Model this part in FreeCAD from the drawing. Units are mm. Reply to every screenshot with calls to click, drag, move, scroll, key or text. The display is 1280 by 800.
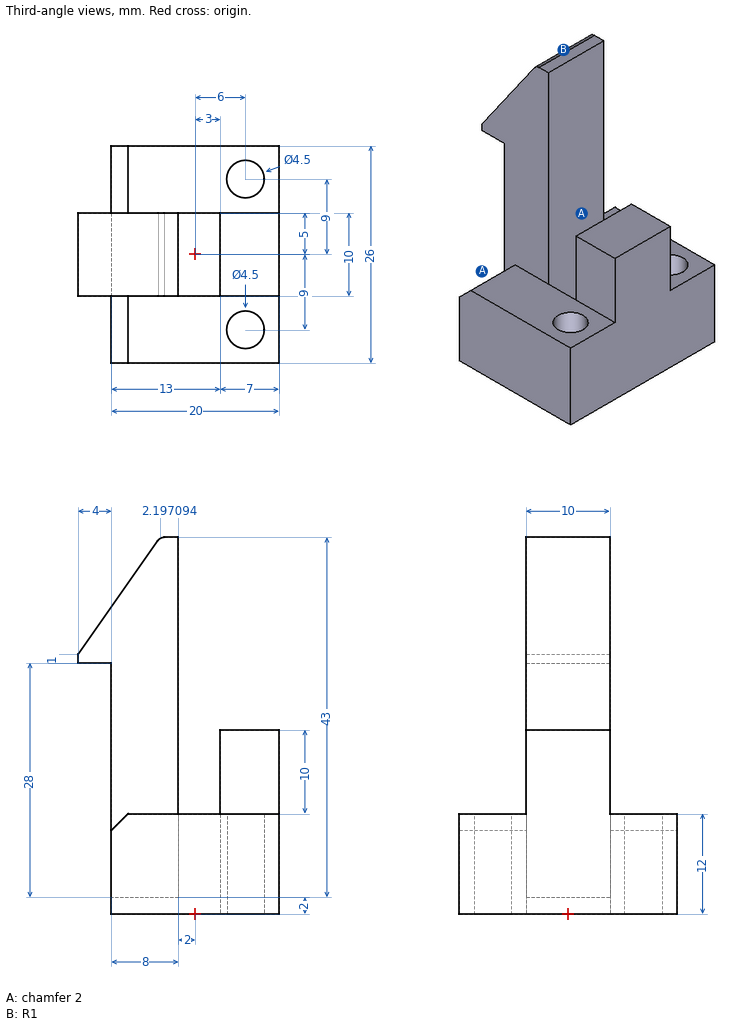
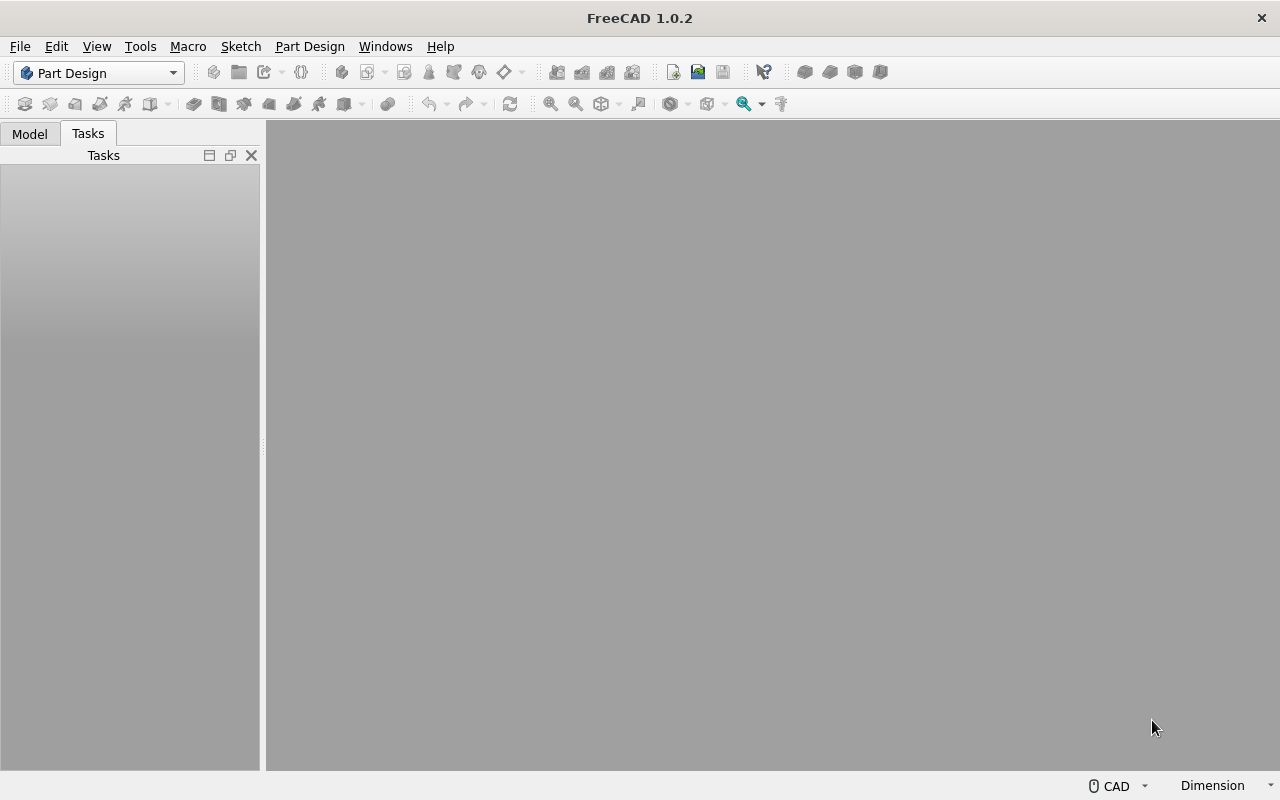
key(ctrl+n)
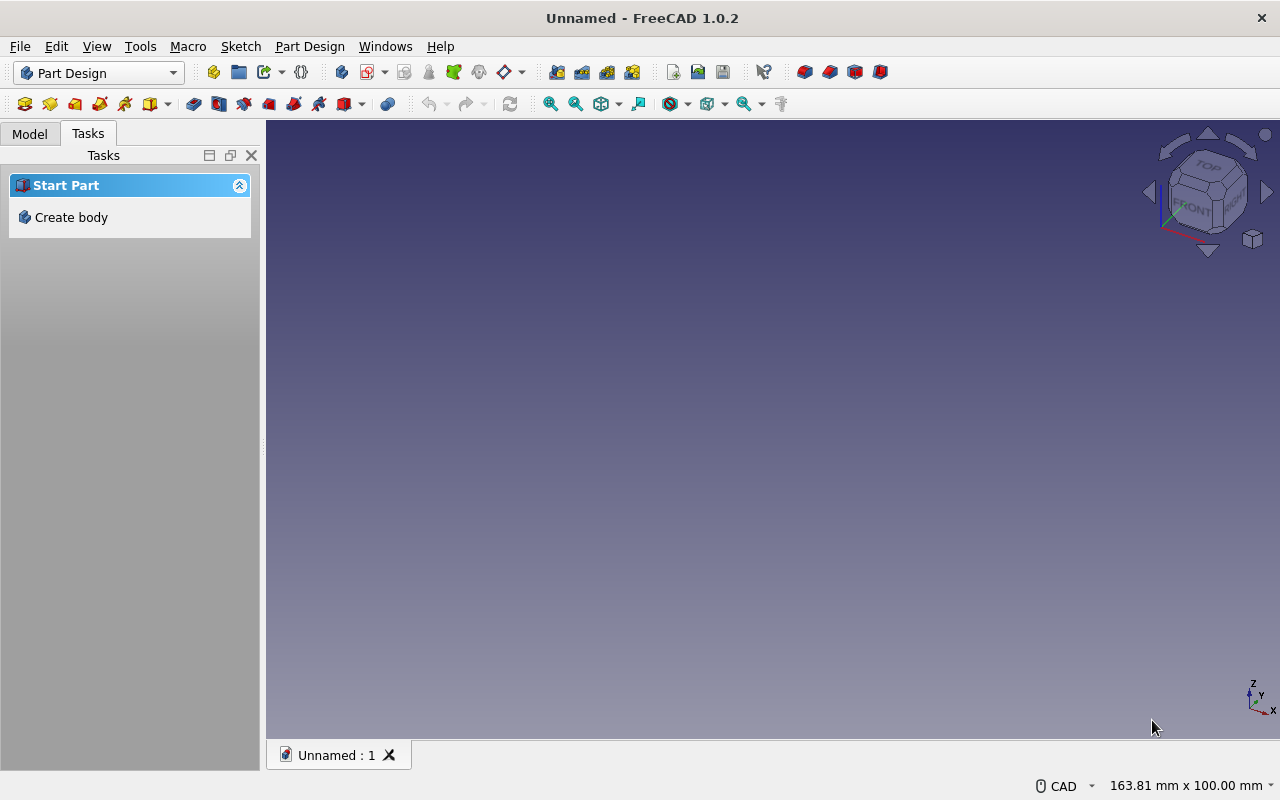
click(366, 72)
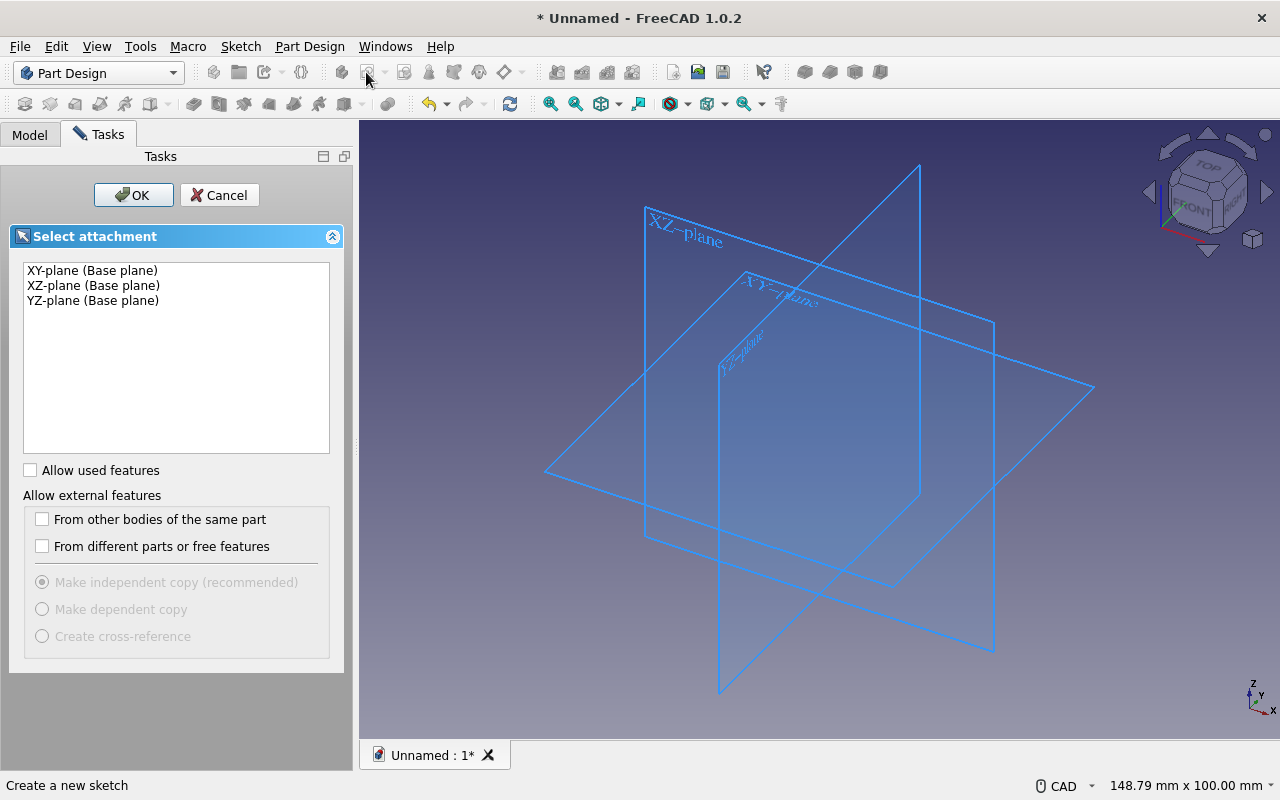
click(84, 270)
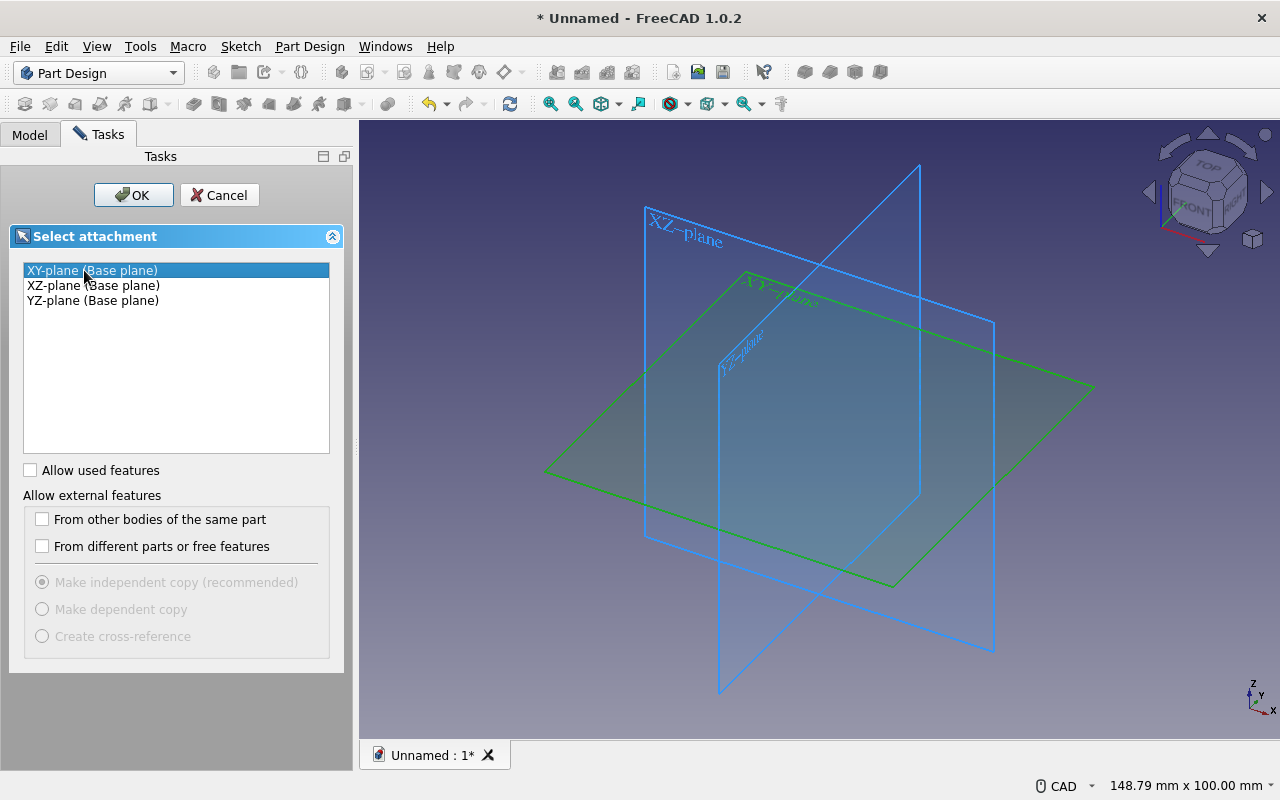
click(134, 195)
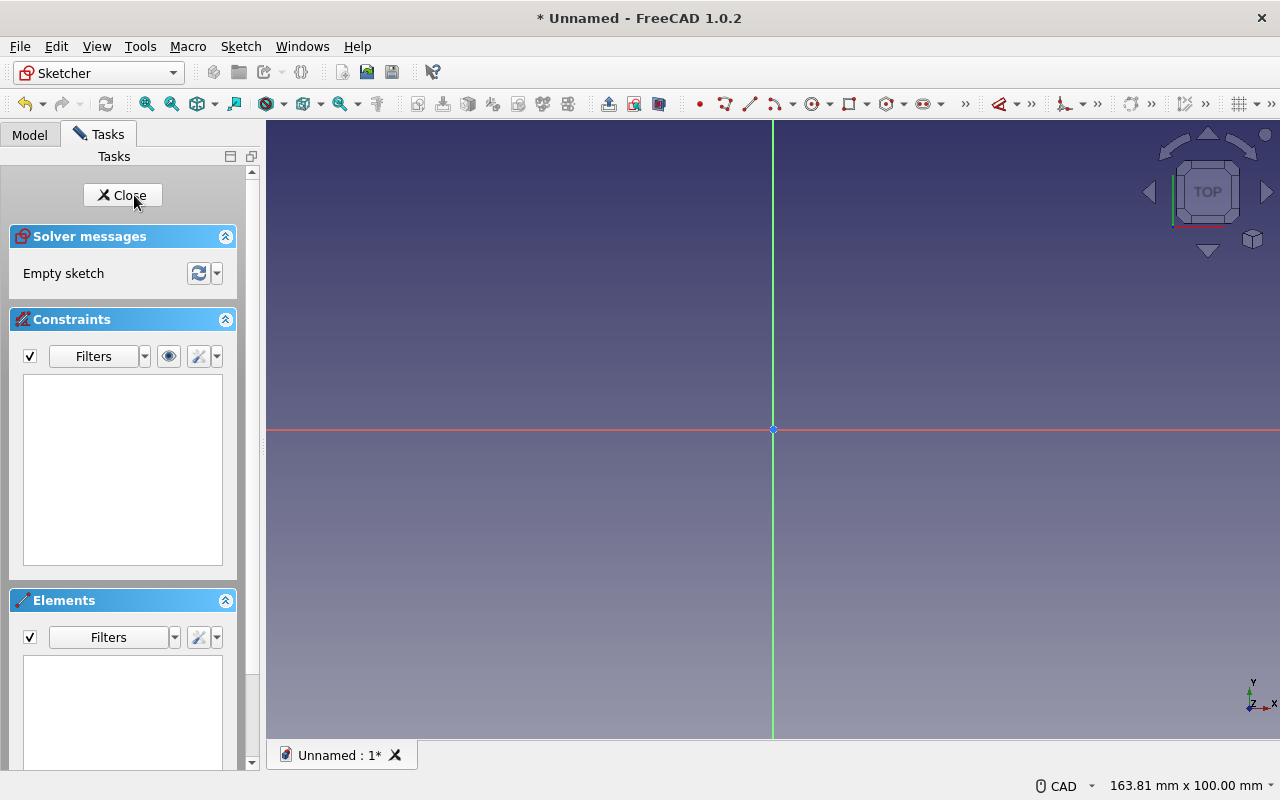
scroll(813, 429, up, 5)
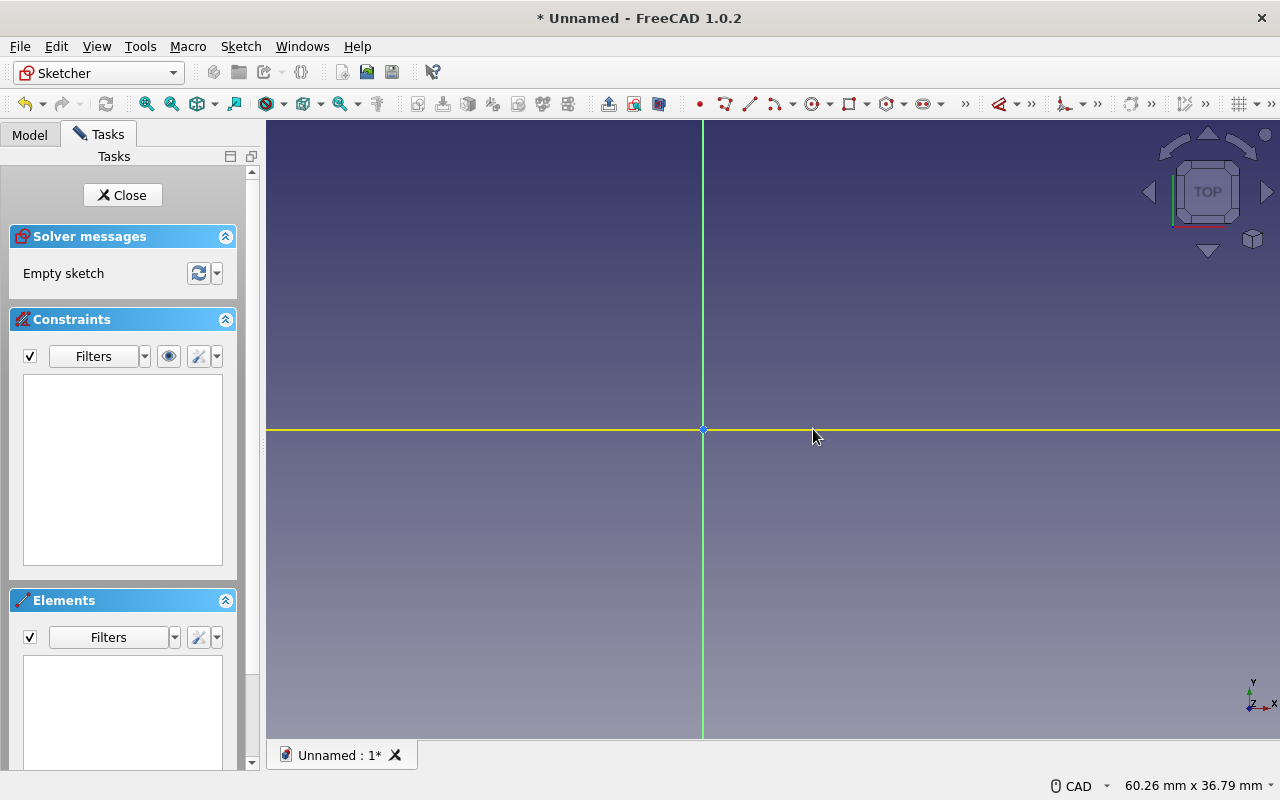
key(g)
key(v)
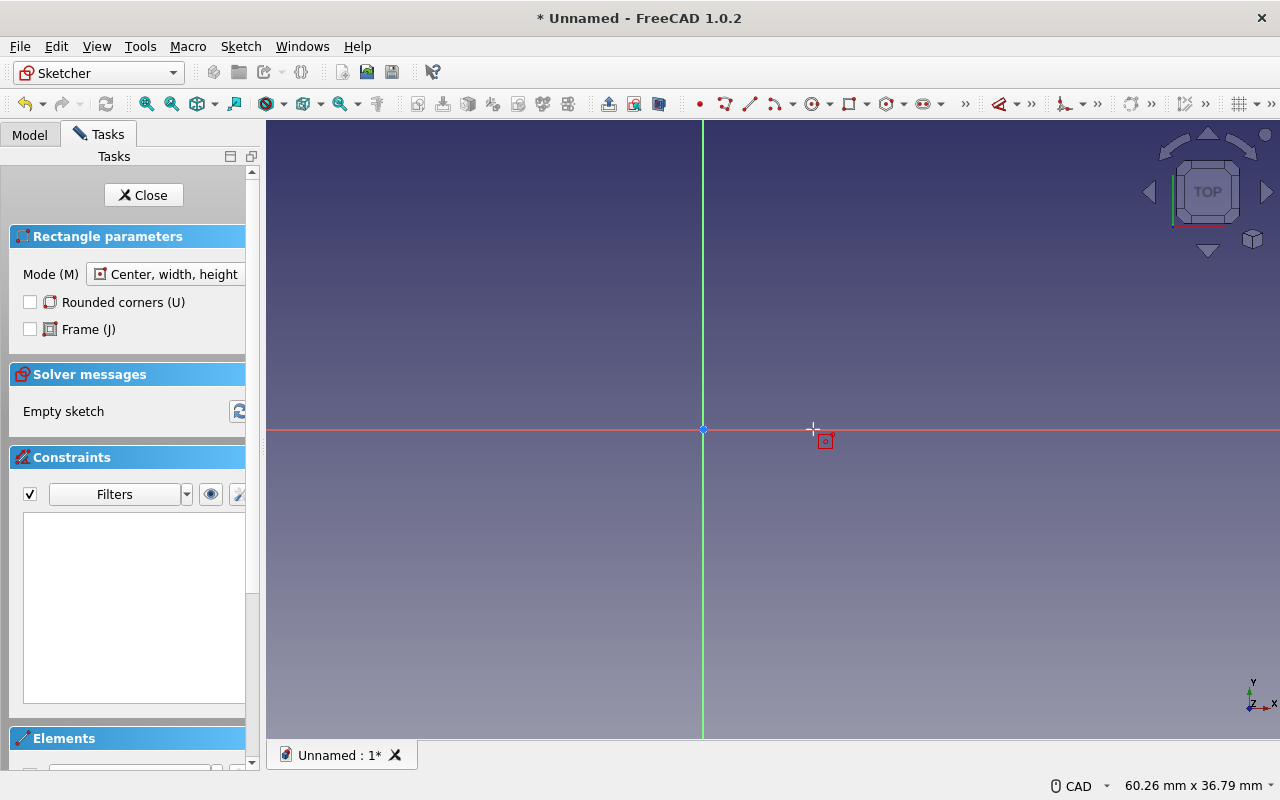
click(703, 430)
click(872, 211)
key(Escape)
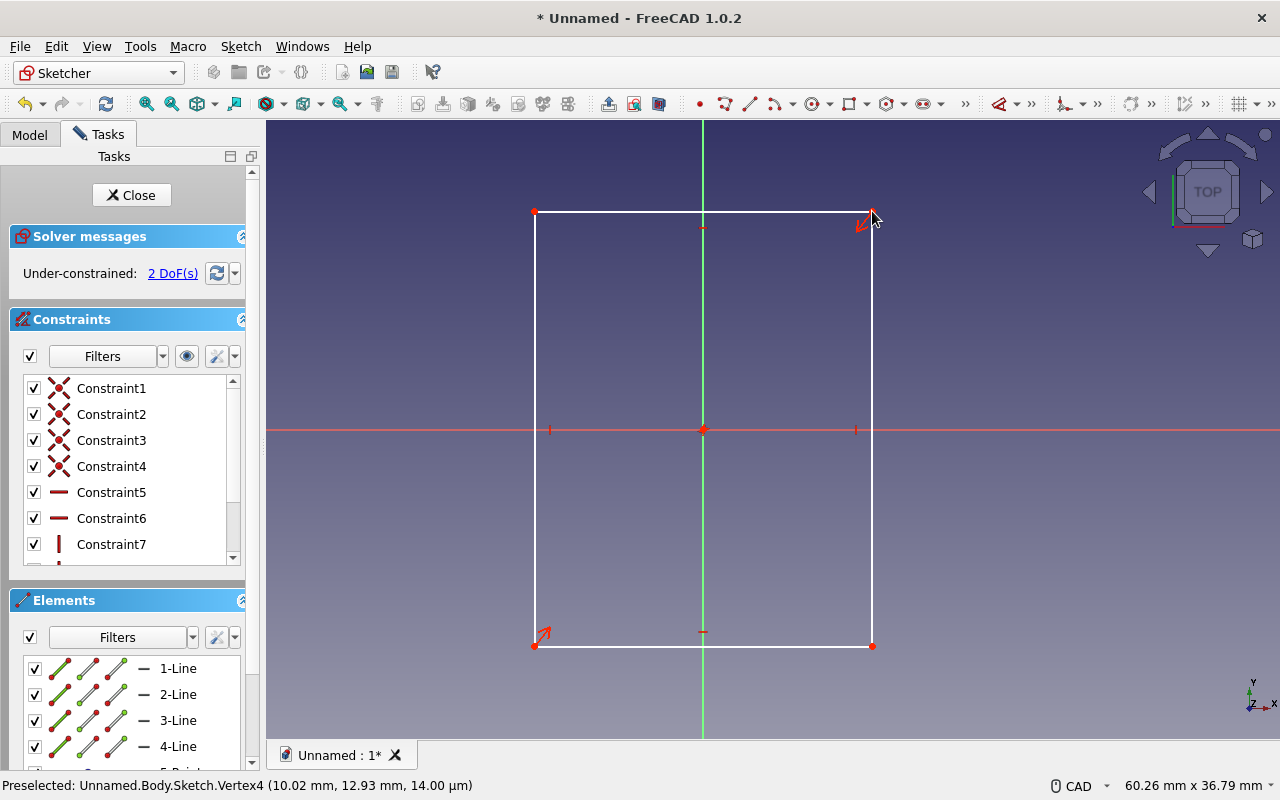
key(d)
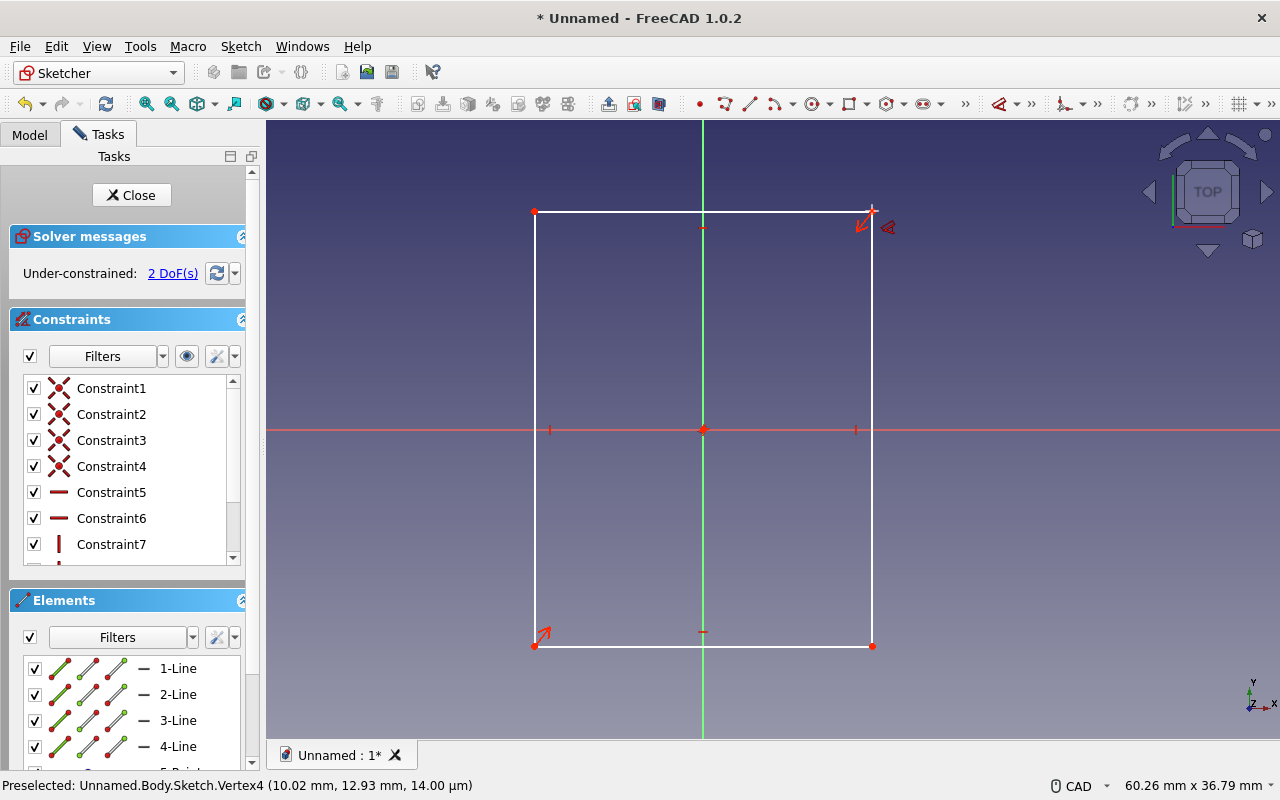
click(636, 647)
click(626, 681)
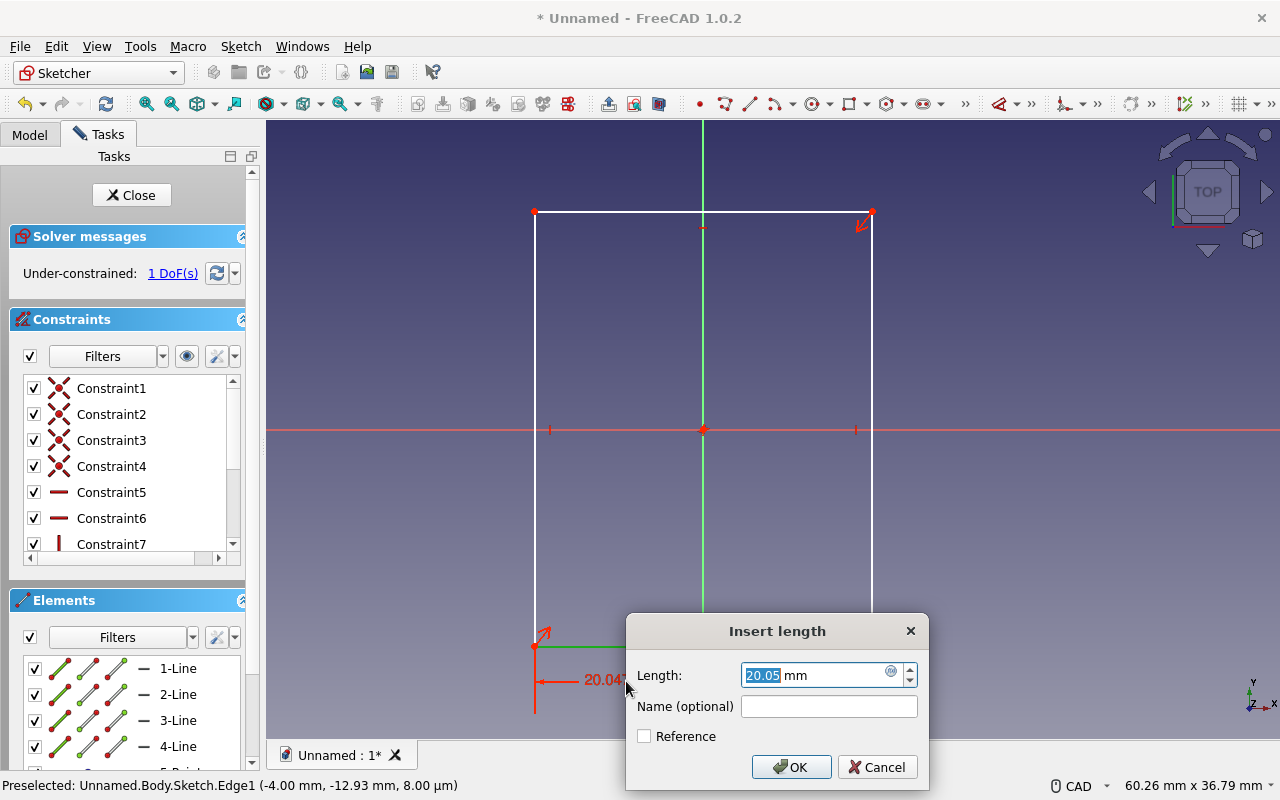
text(20)
key(Return)